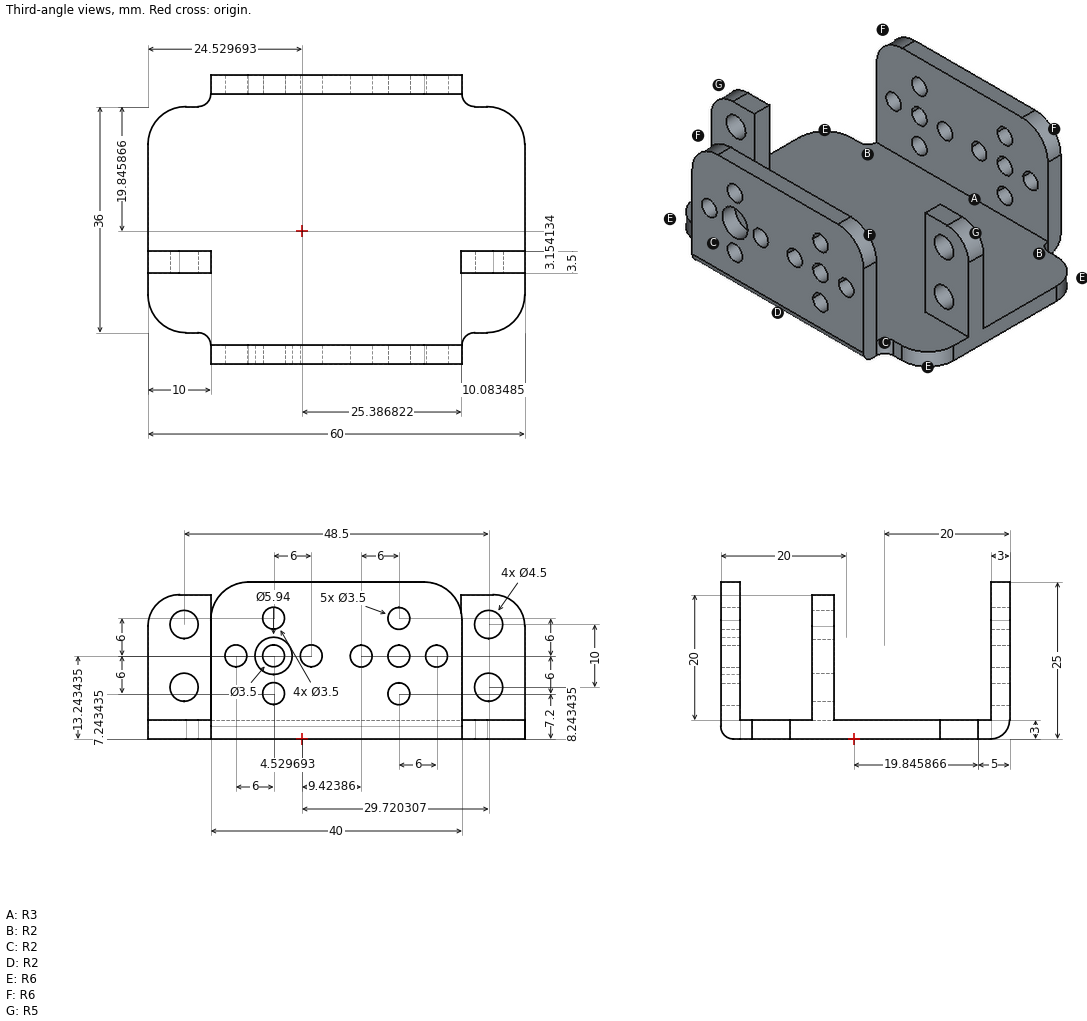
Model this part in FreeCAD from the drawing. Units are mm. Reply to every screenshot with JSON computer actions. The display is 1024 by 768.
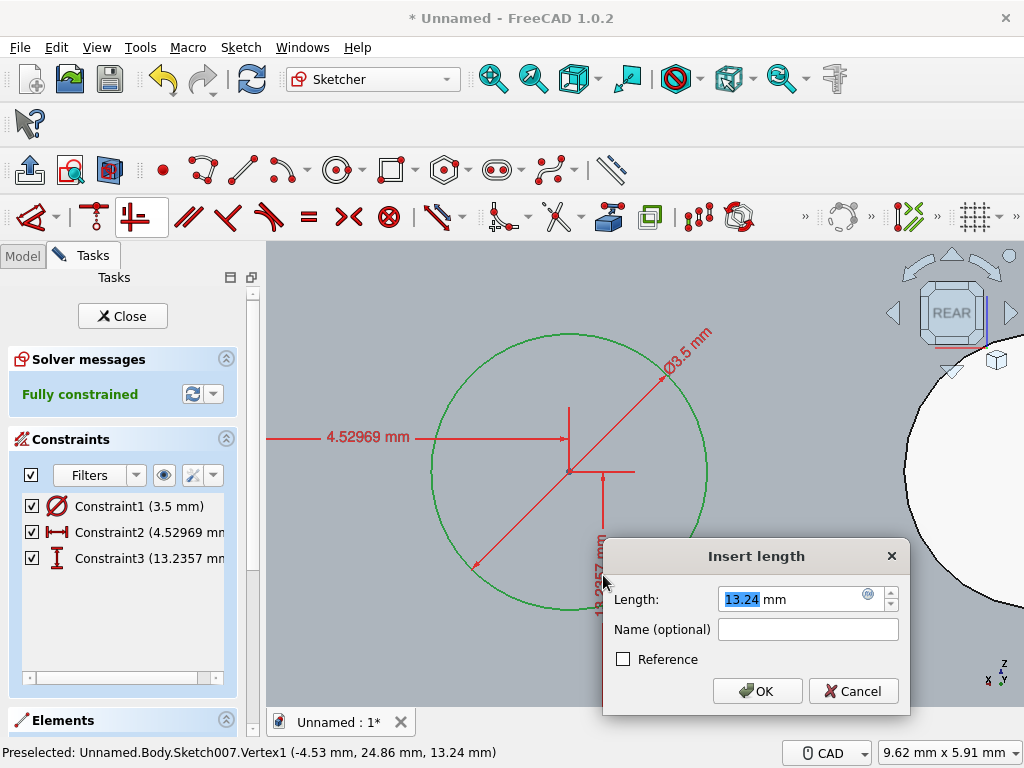
{"action": "type", "text": "13.243435"}
{"action": "key", "text": "Return"}
{"action": "key", "text": "Escape"}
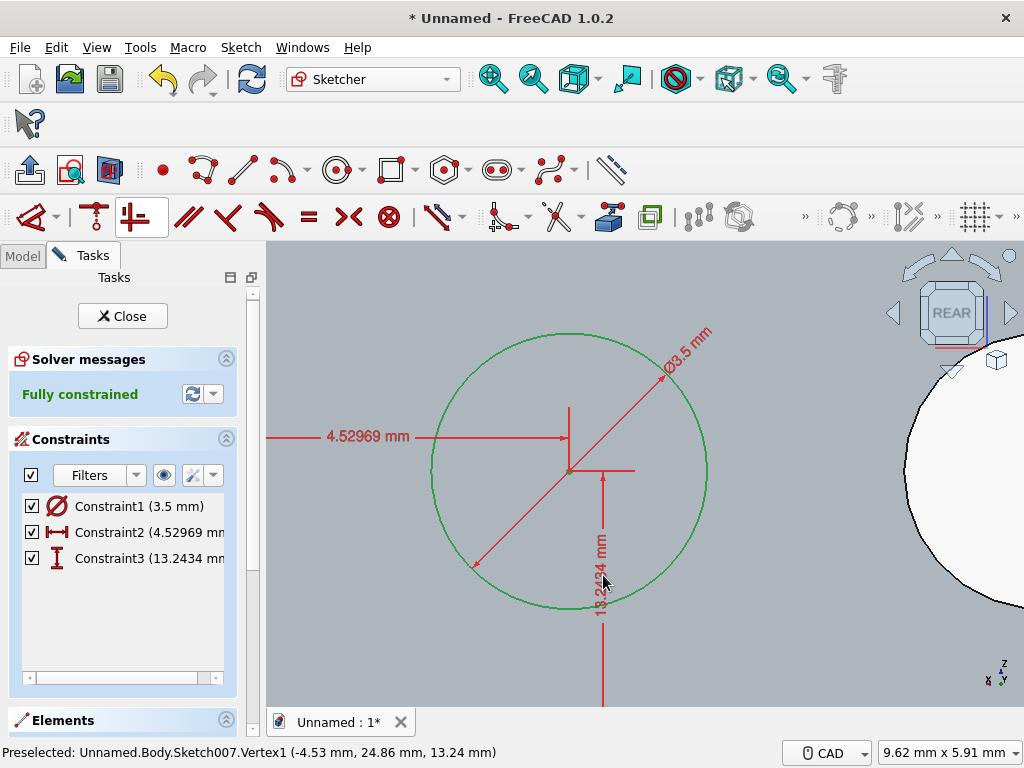
{"action": "left_click", "coordinate": [123, 316]}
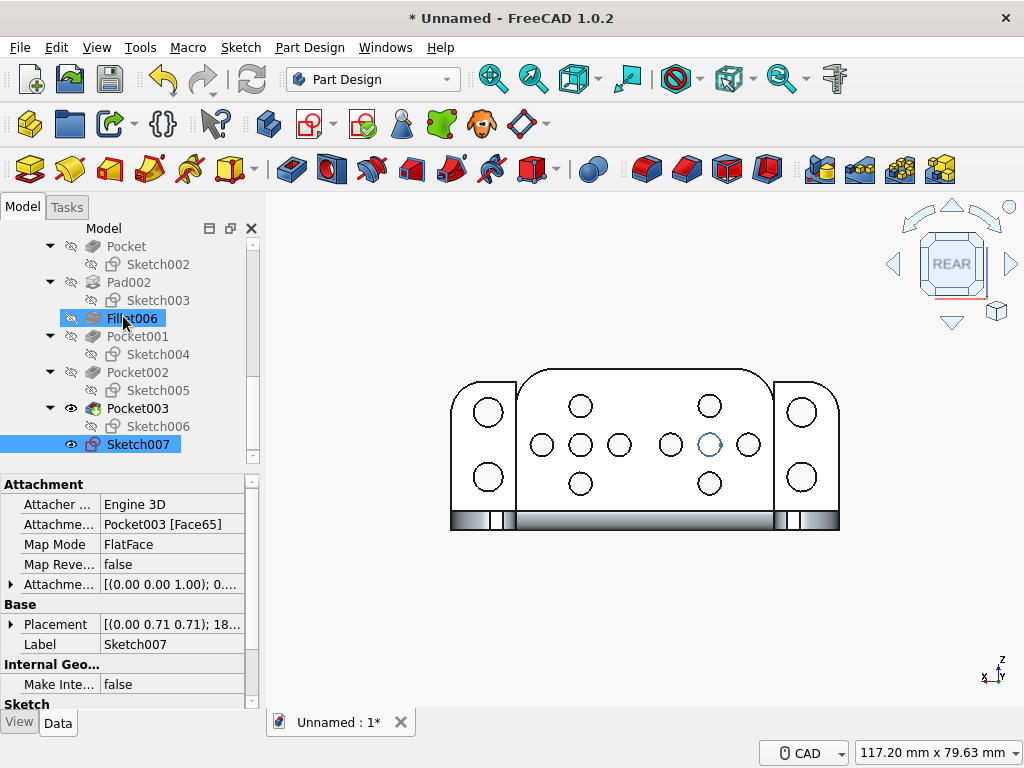
{"action": "left_click", "coordinate": [292, 170]}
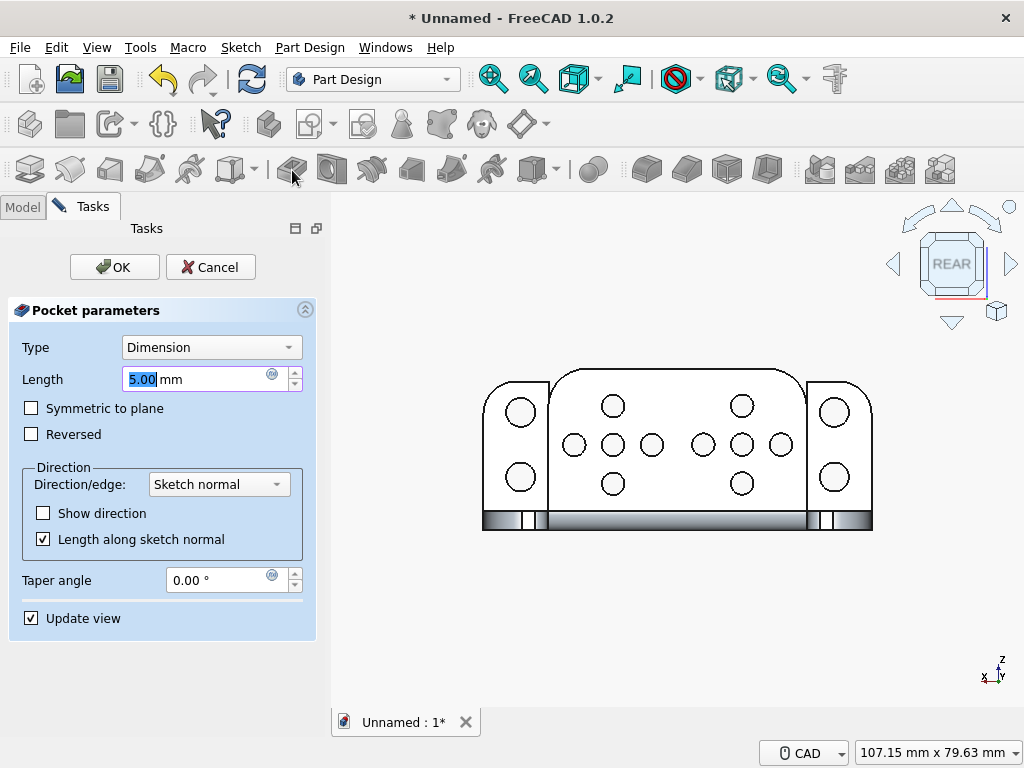
{"action": "type", "text": "20"}
{"action": "key", "text": "Tab"}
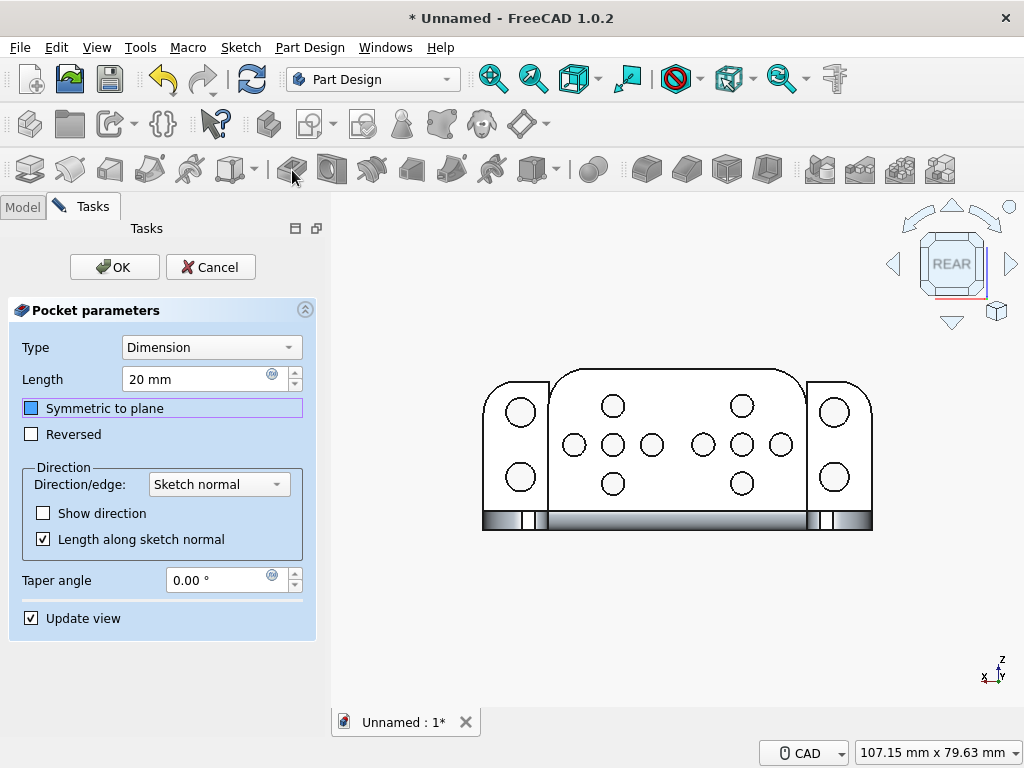
{"action": "left_click", "coordinate": [115, 267]}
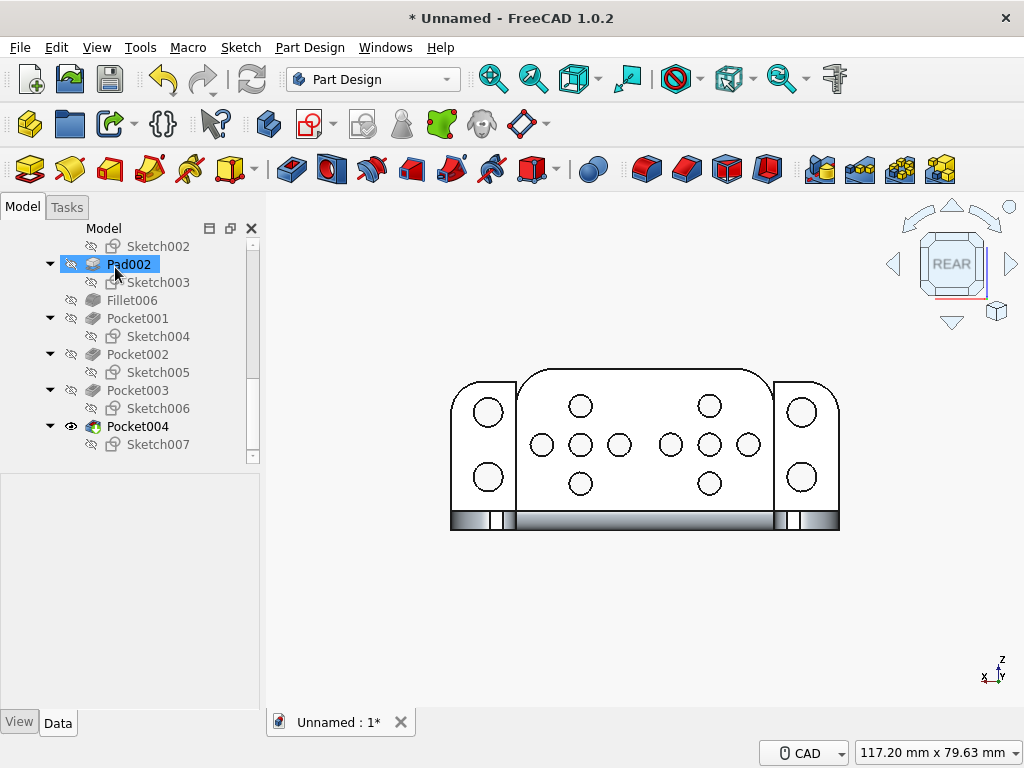
{"action": "key", "text": "0"}